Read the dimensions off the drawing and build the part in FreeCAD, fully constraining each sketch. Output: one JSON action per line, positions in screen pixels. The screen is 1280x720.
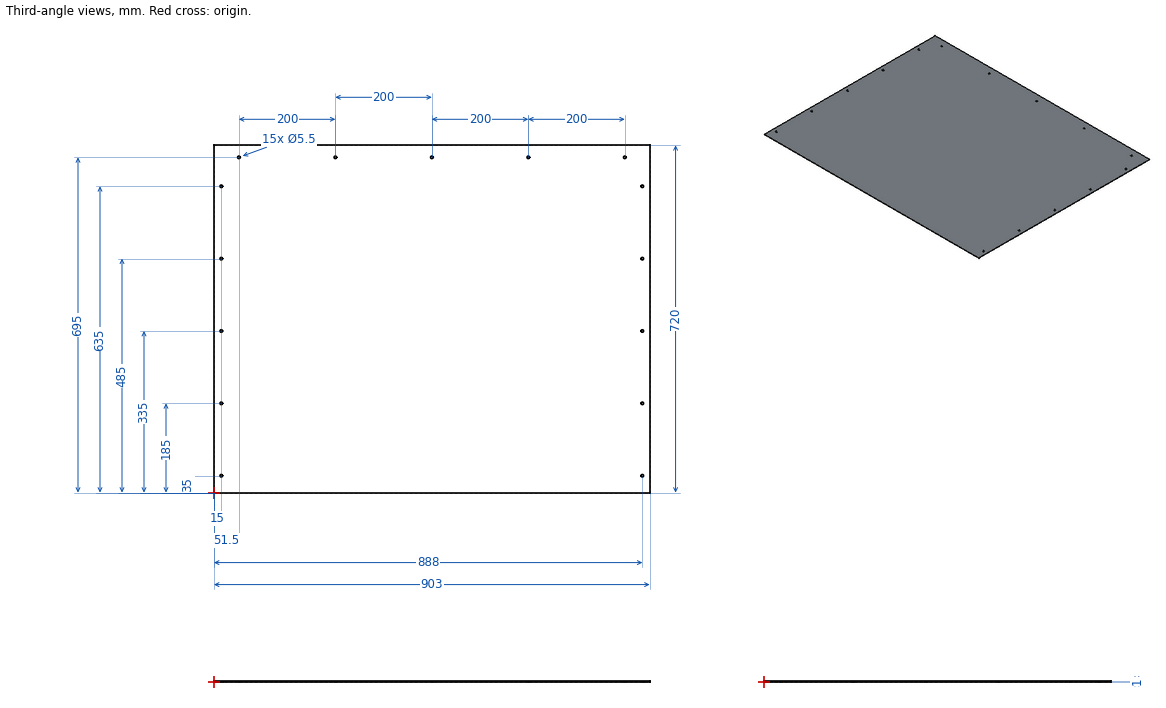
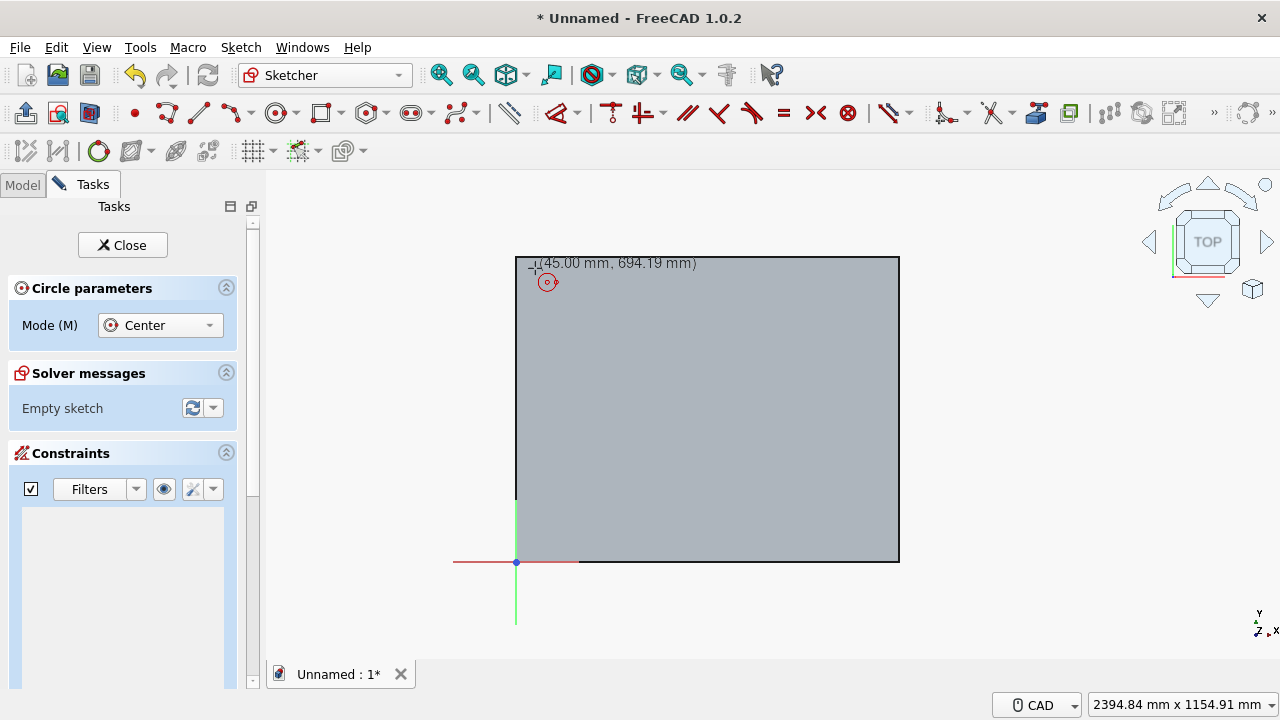
{"action": "left_click", "coordinate": [538, 268]}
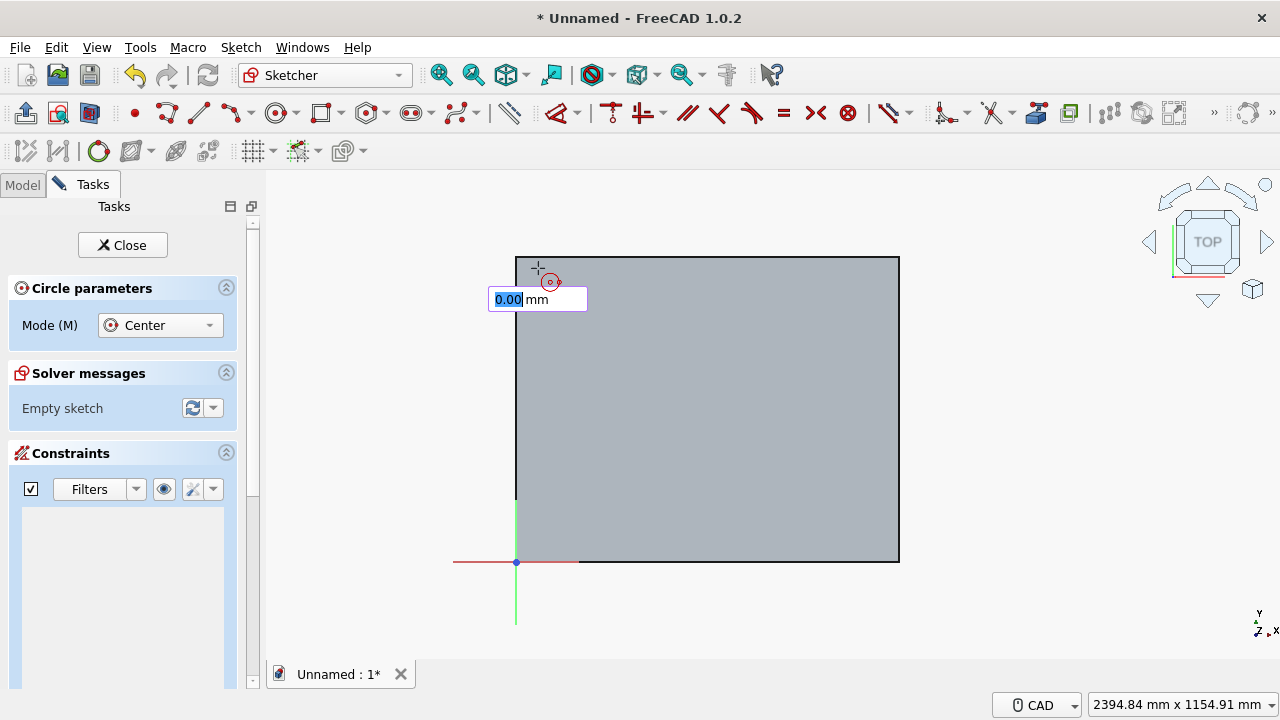
{"action": "scroll", "coordinate": [539, 267], "scroll_direction": "up", "scroll_amount": 14}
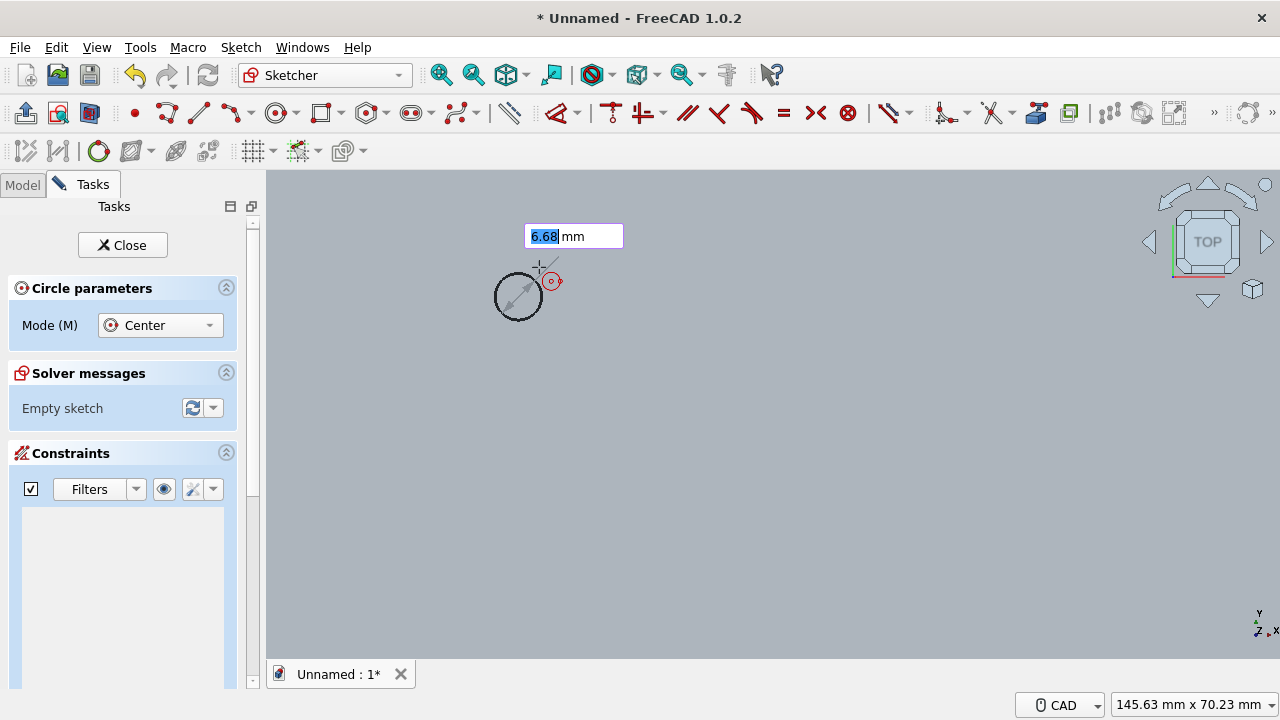
{"action": "left_click", "coordinate": [532, 265]}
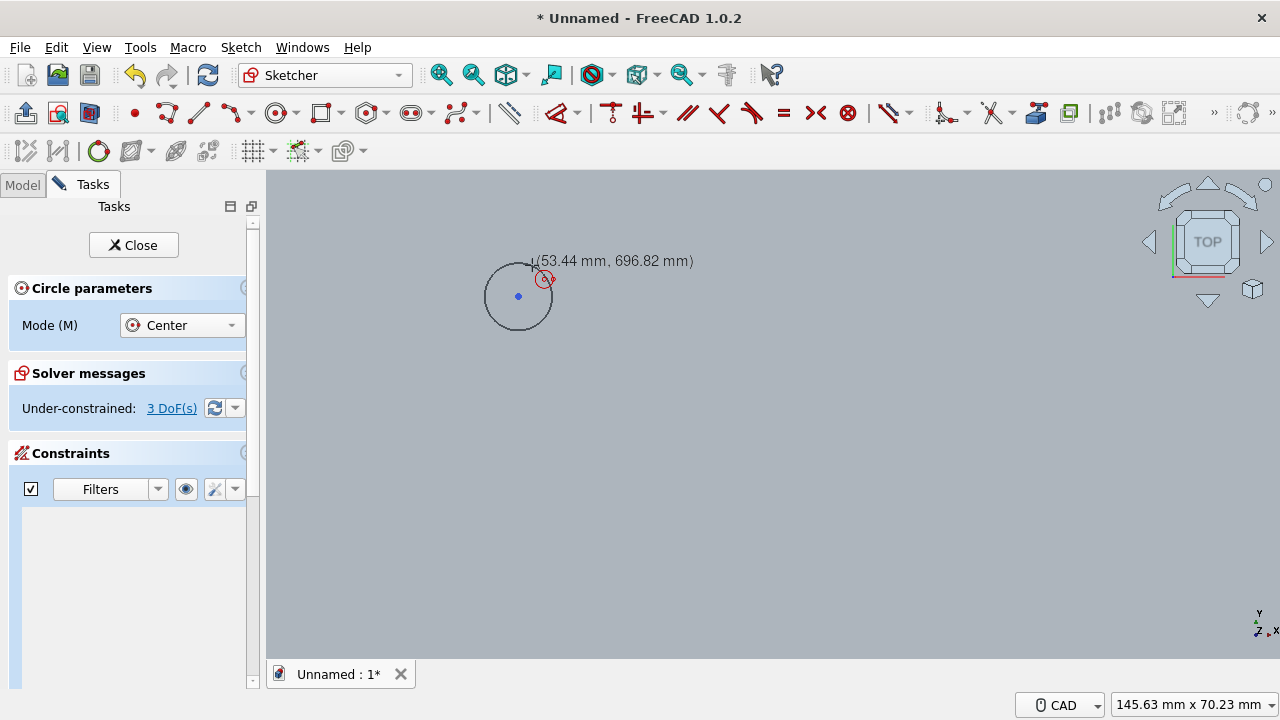
{"action": "scroll", "coordinate": [539, 267], "scroll_direction": "down", "scroll_amount": 14}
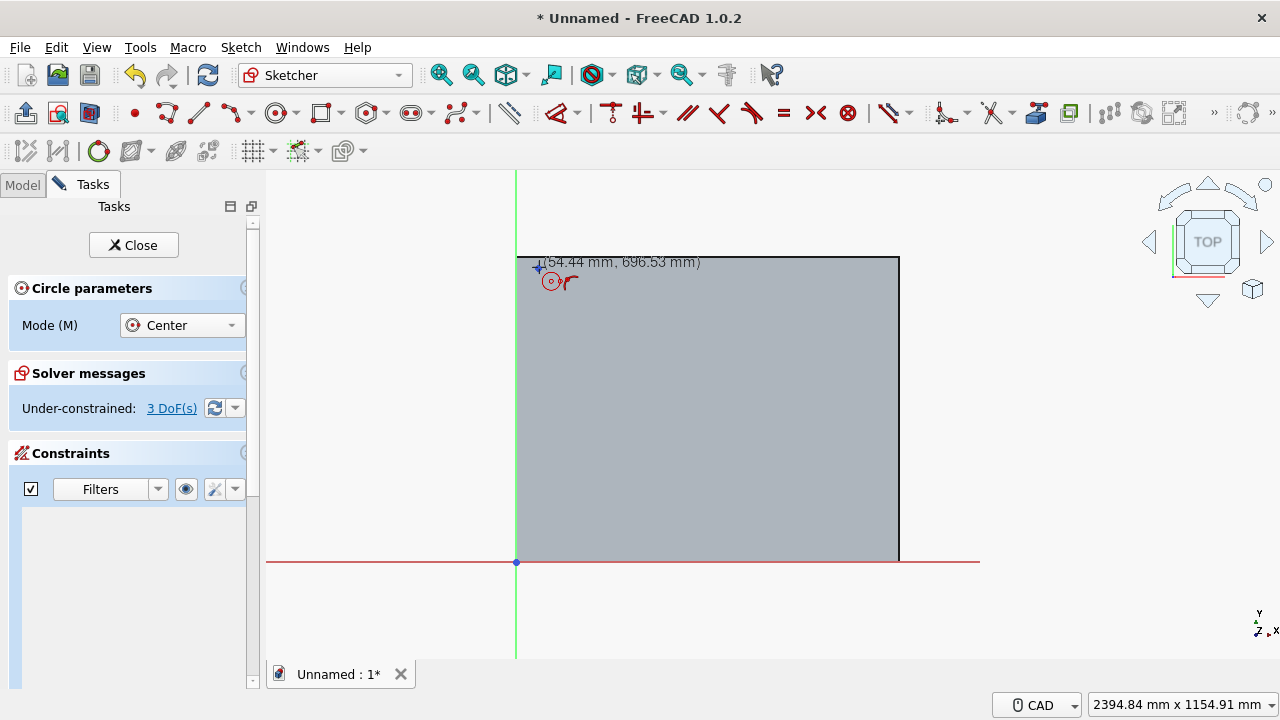
{"action": "scroll", "coordinate": [523, 293], "scroll_direction": "up", "scroll_amount": 15}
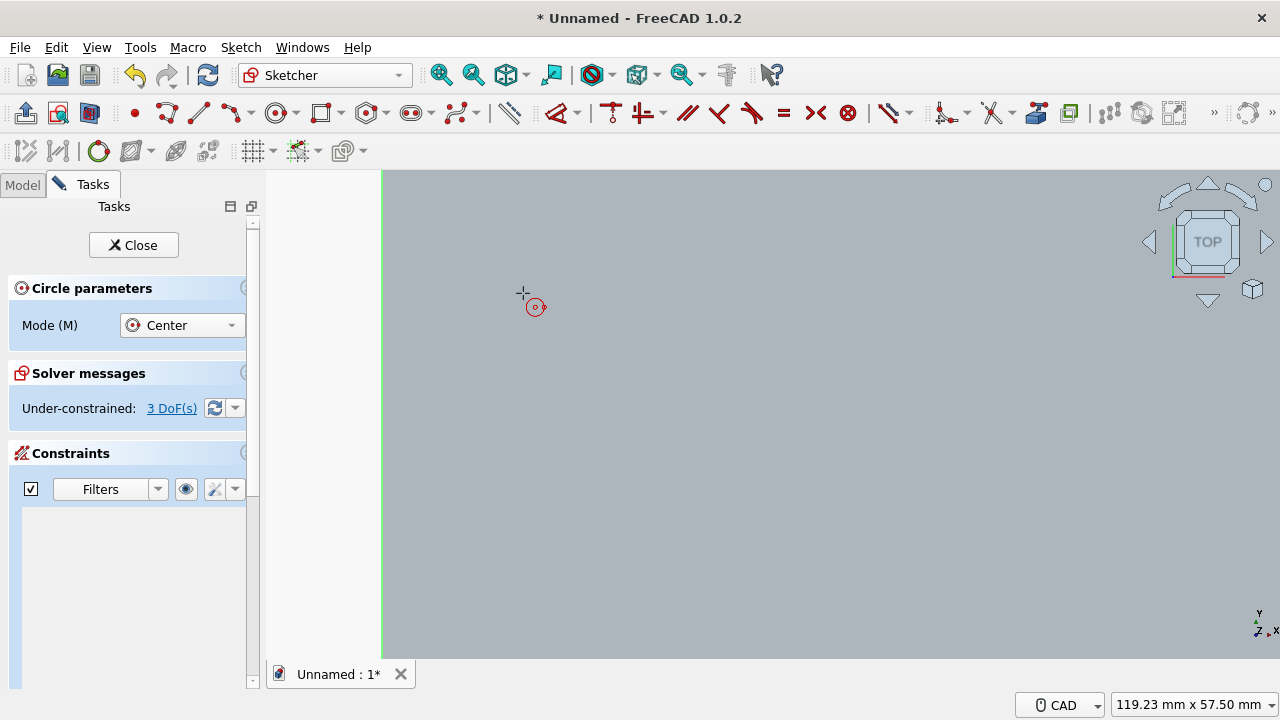
{"action": "scroll", "coordinate": [523, 293], "scroll_direction": "down", "scroll_amount": 15}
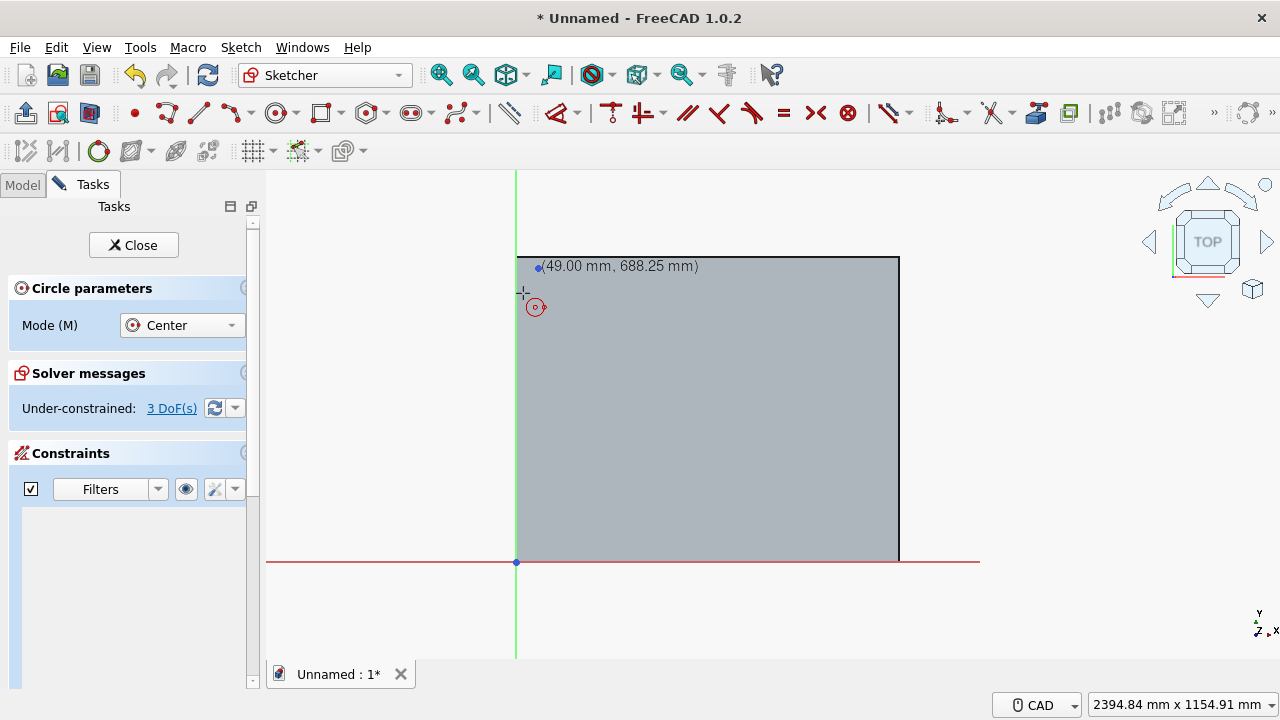
{"action": "scroll", "coordinate": [523, 293], "scroll_direction": "up", "scroll_amount": 5}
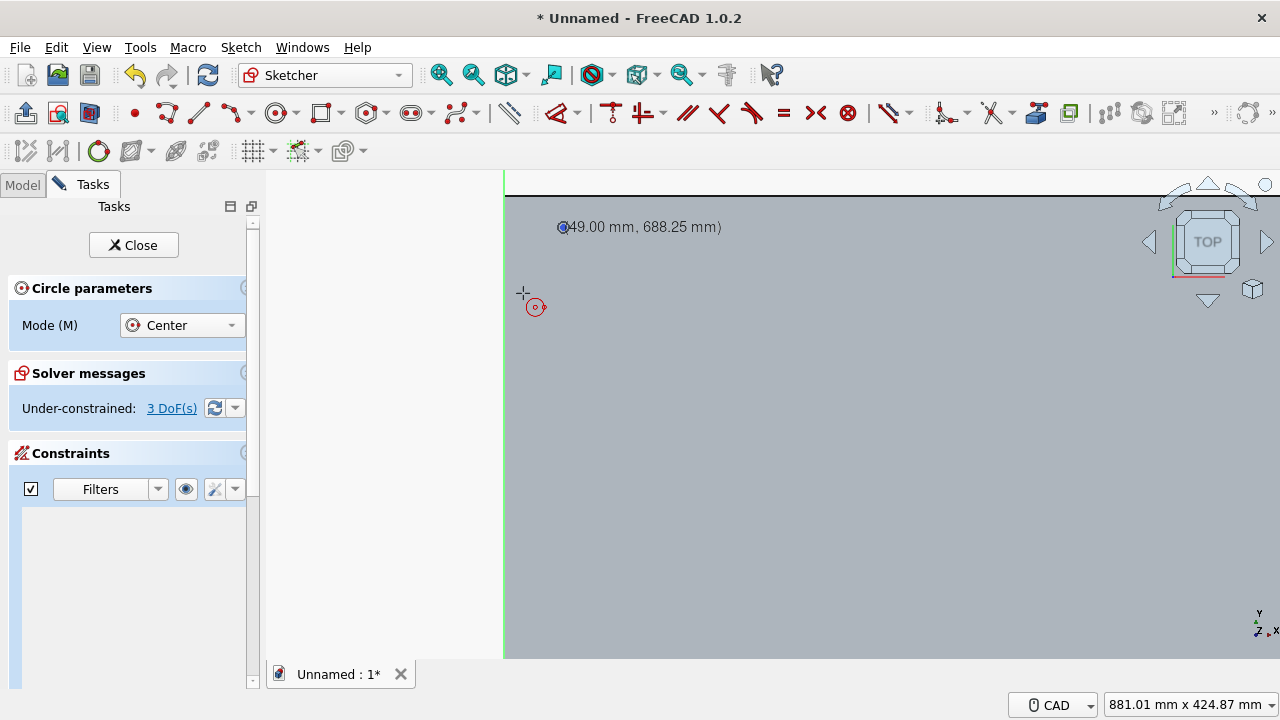
{"action": "left_click", "coordinate": [521, 293]}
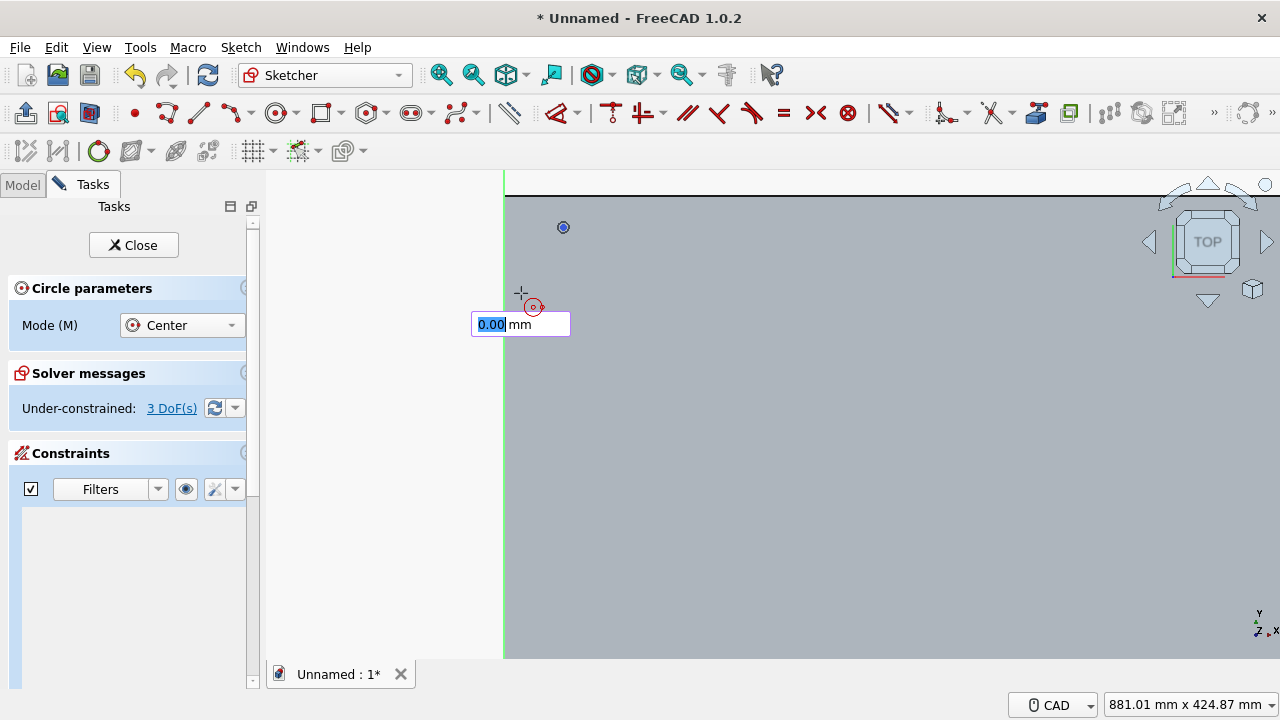
{"action": "scroll", "coordinate": [524, 291], "scroll_direction": "up", "scroll_amount": 9}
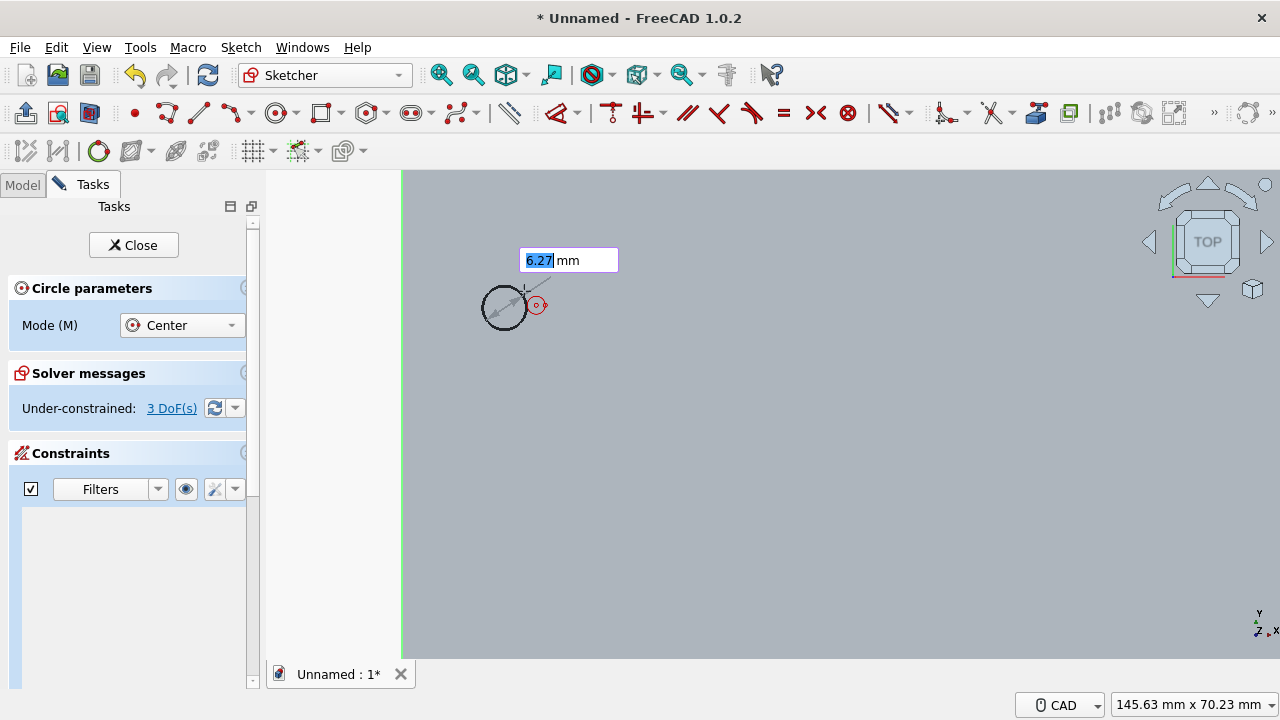
{"action": "left_click", "coordinate": [520, 291]}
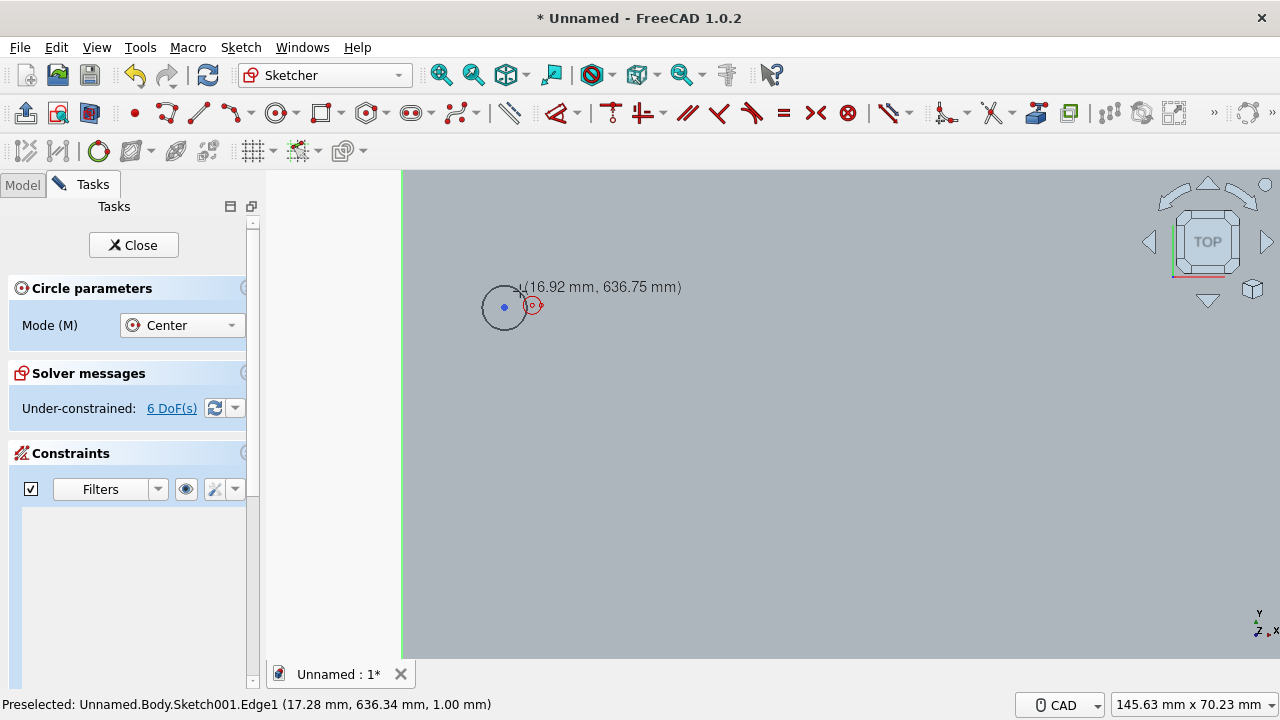
{"action": "scroll", "coordinate": [523, 293], "scroll_direction": "down", "scroll_amount": 14}